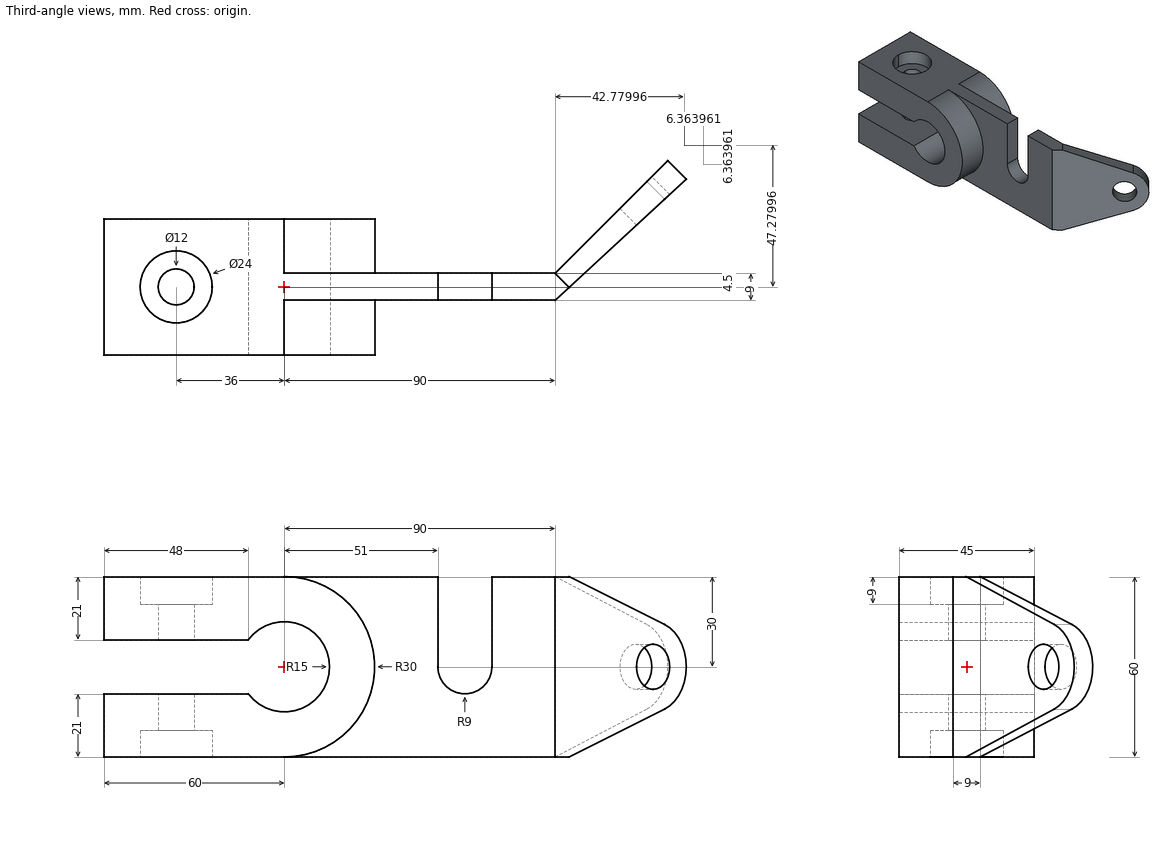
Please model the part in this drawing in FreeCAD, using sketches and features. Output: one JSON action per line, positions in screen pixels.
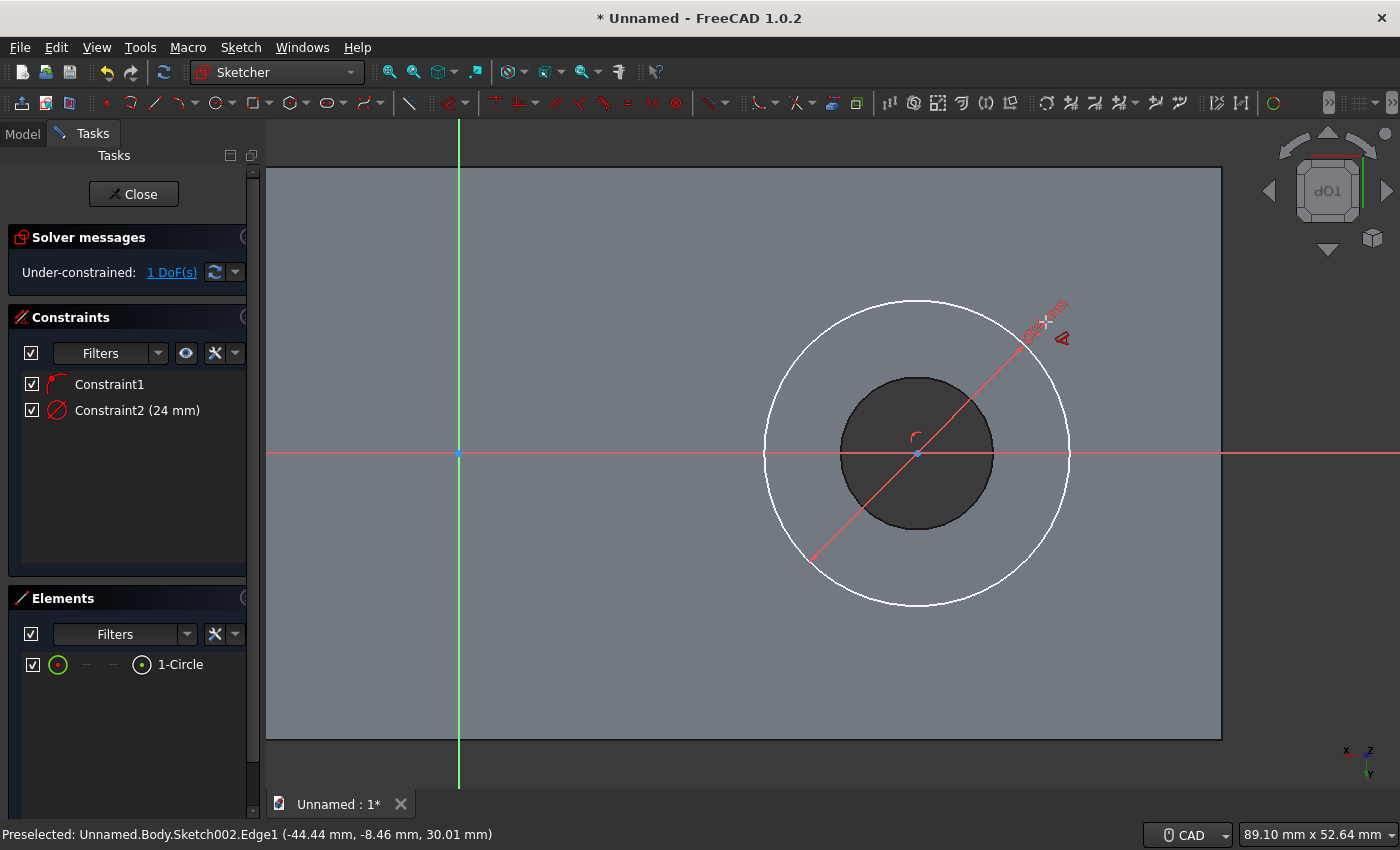
{"action": "left_click", "coordinate": [917, 453]}
{"action": "left_click", "coordinate": [688, 487]}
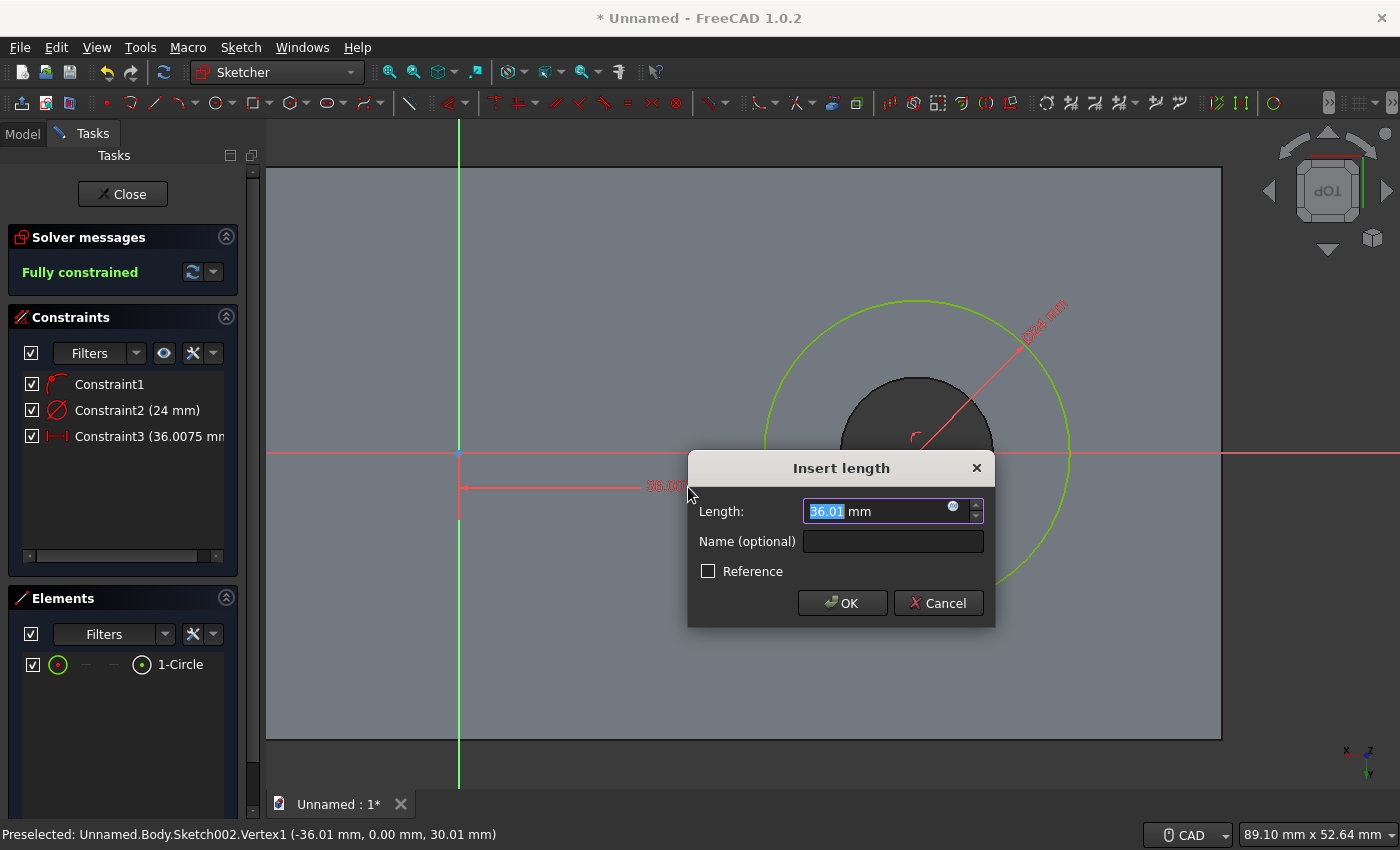
{"action": "type", "text": "36"}
{"action": "key", "text": "Return"}
{"action": "key", "text": "Escape"}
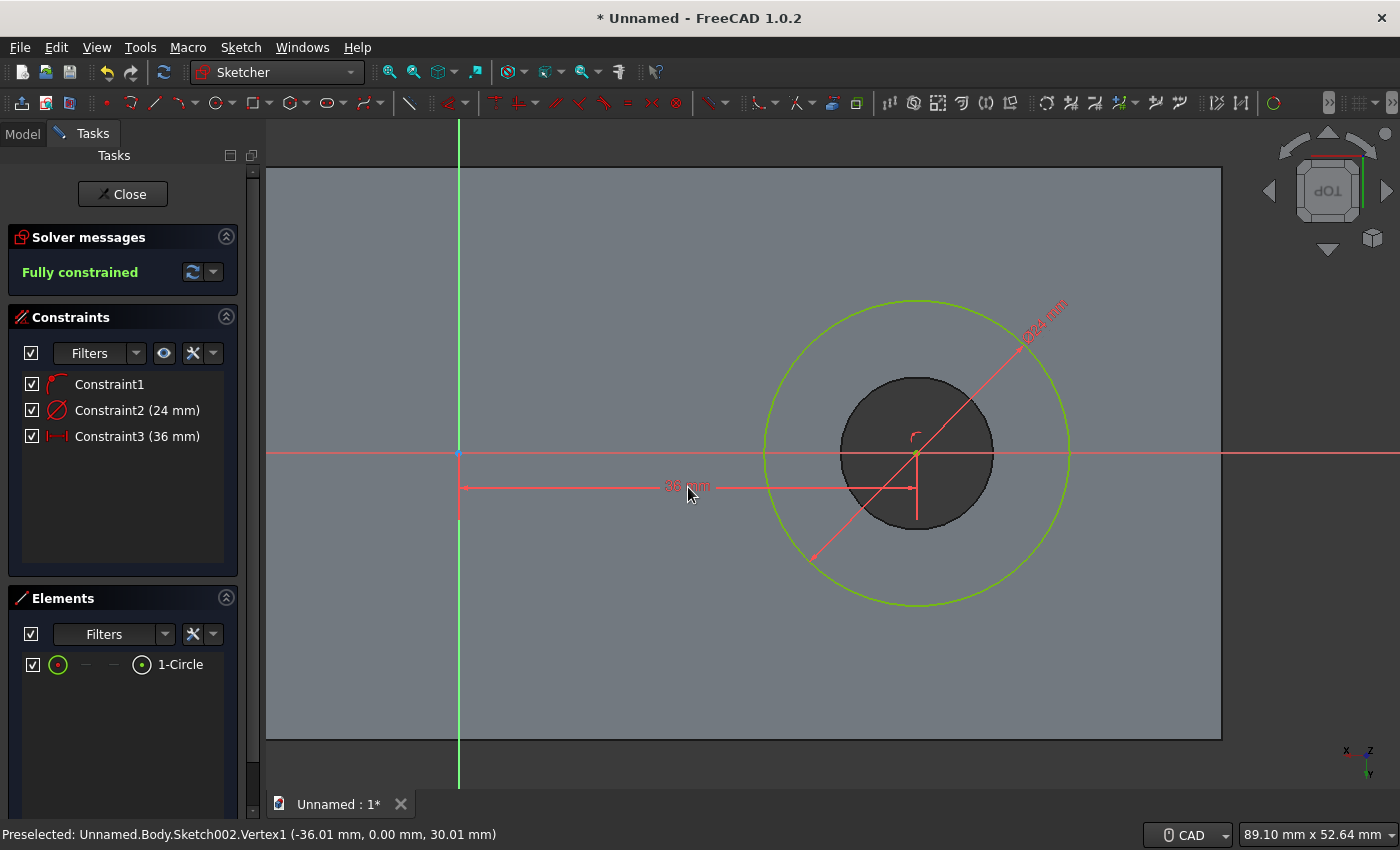
{"action": "left_click", "coordinate": [123, 194]}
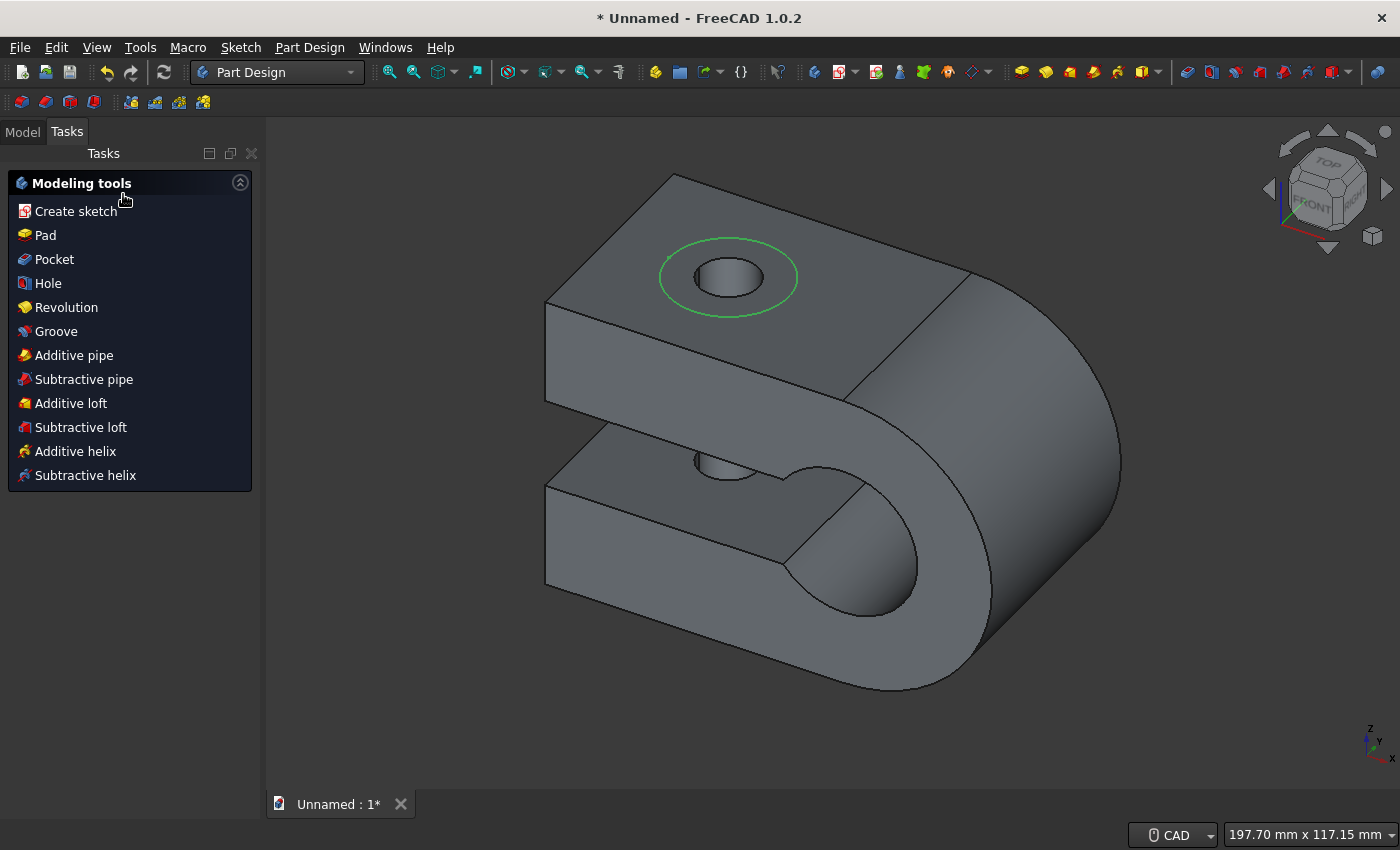
{"action": "left_click", "coordinate": [1188, 72]}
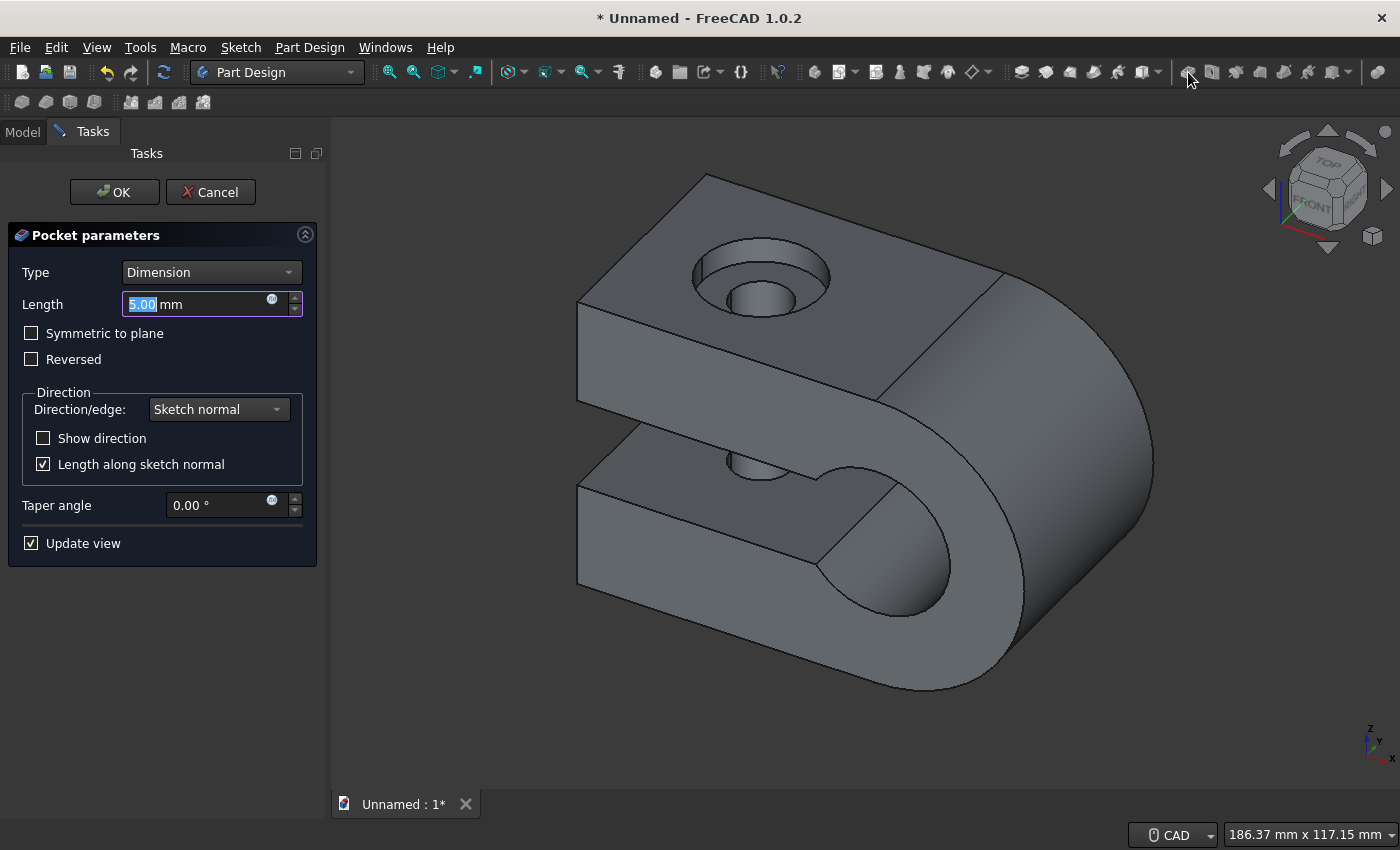
{"action": "type", "text": "9"}
{"action": "key", "text": "Tab"}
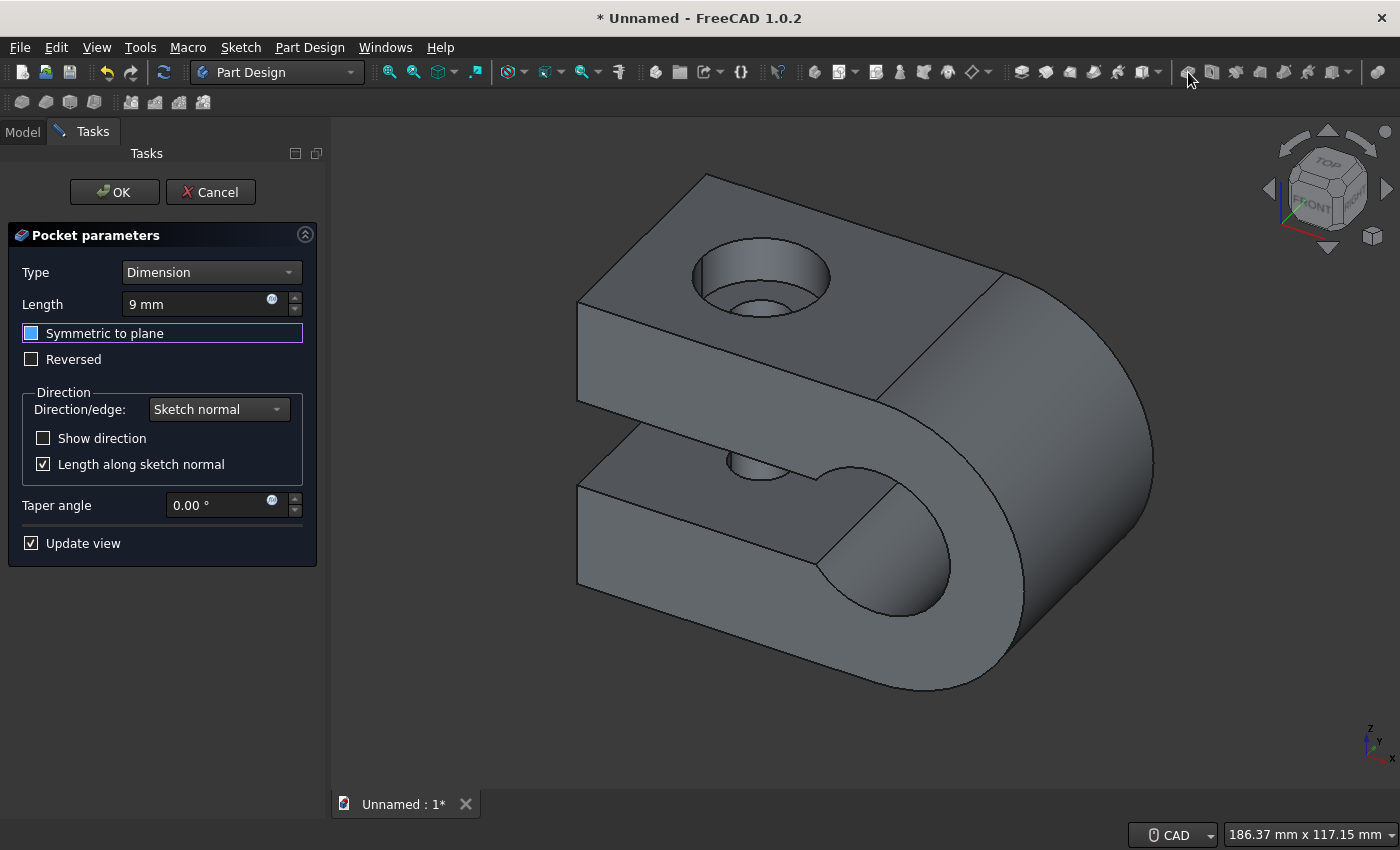
{"action": "left_click", "coordinate": [115, 192]}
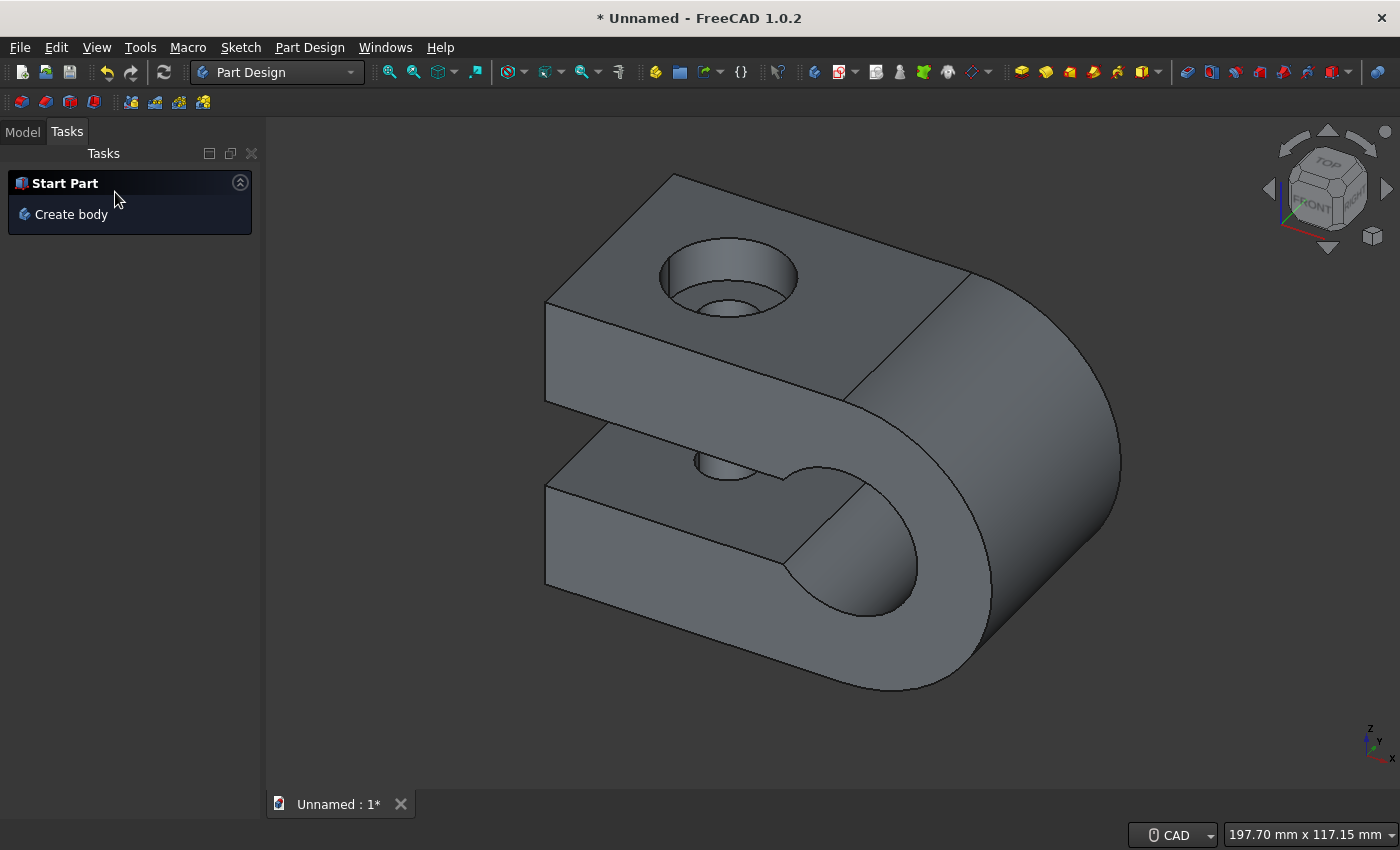
{"action": "left_click", "coordinate": [23, 131]}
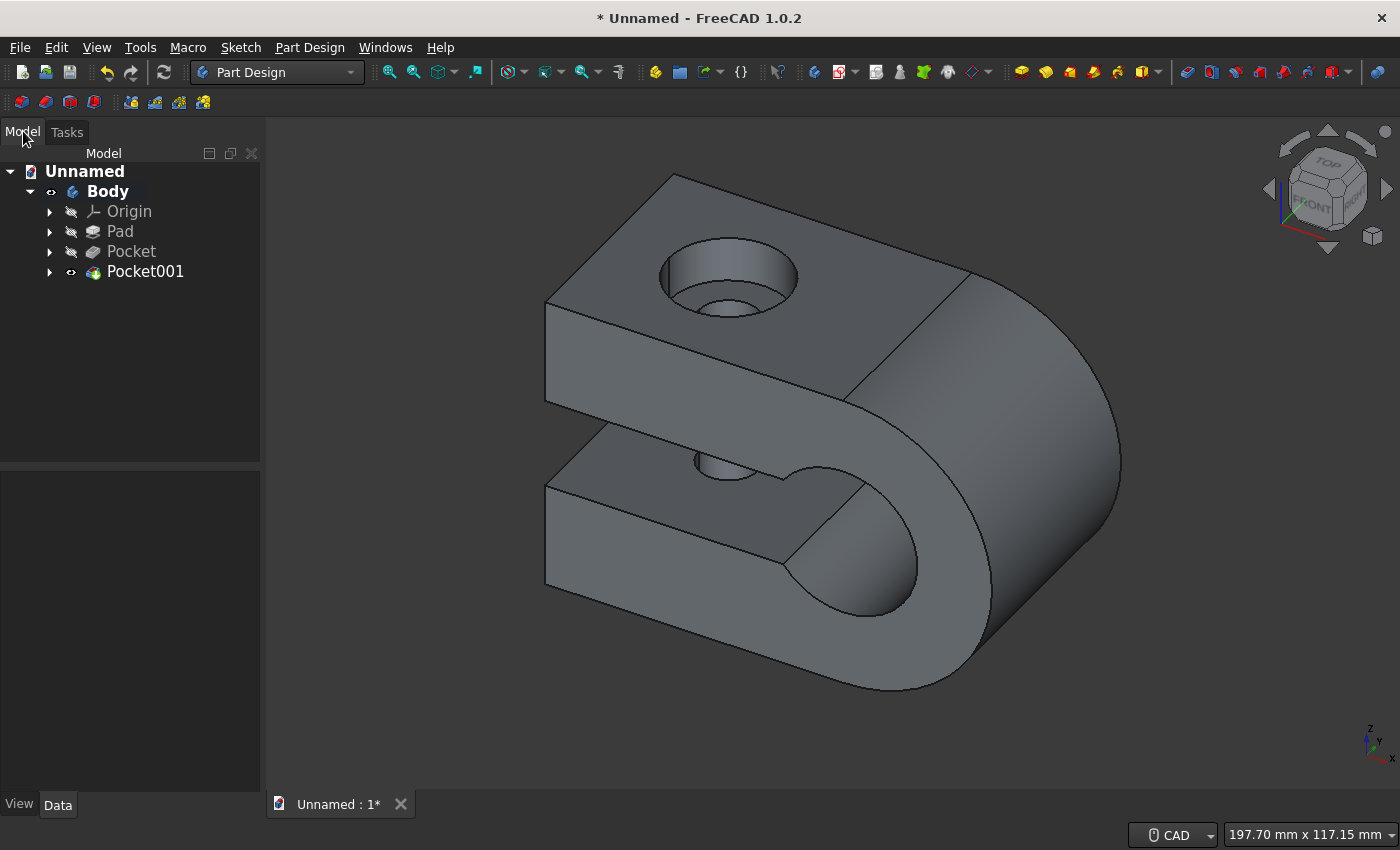
{"action": "left_click", "coordinate": [116, 272]}